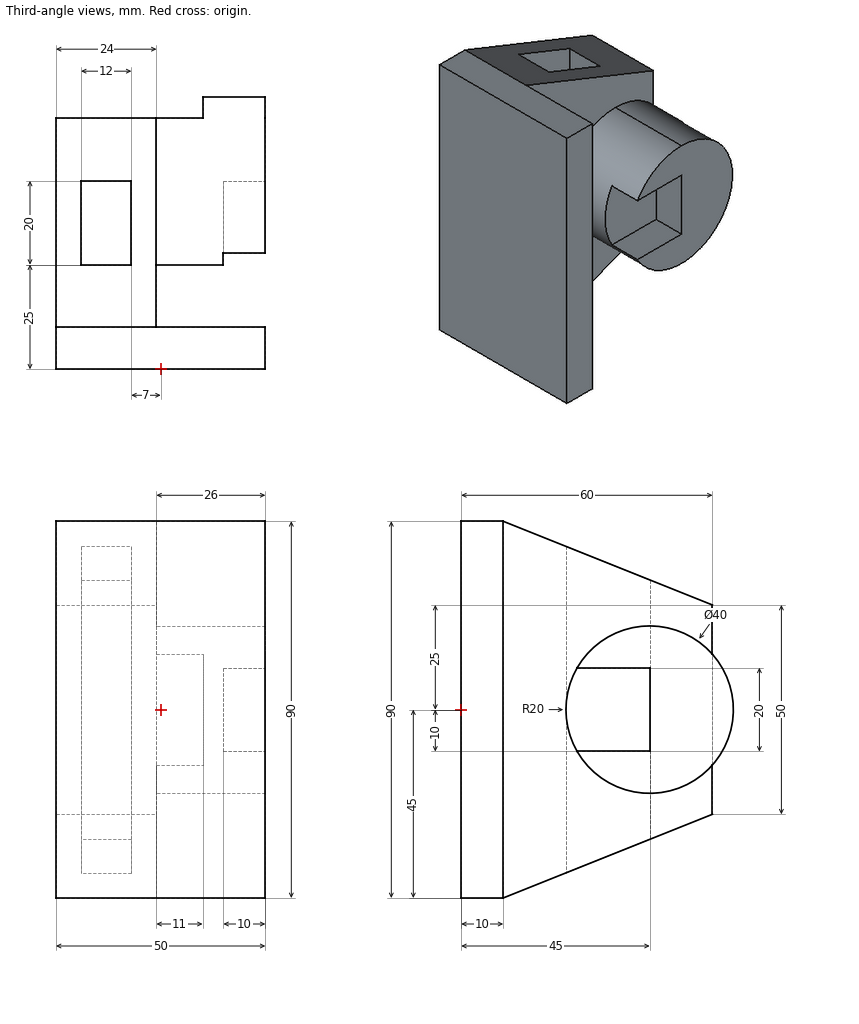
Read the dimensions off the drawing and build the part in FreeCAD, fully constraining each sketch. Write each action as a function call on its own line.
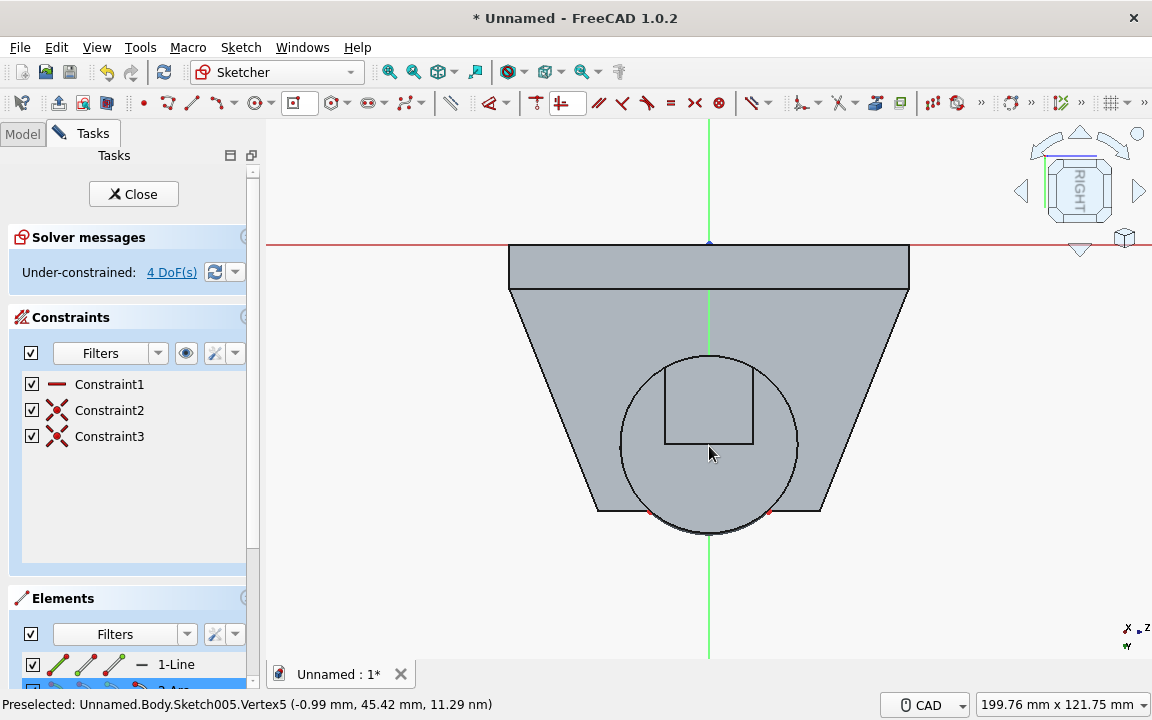
click(709, 596)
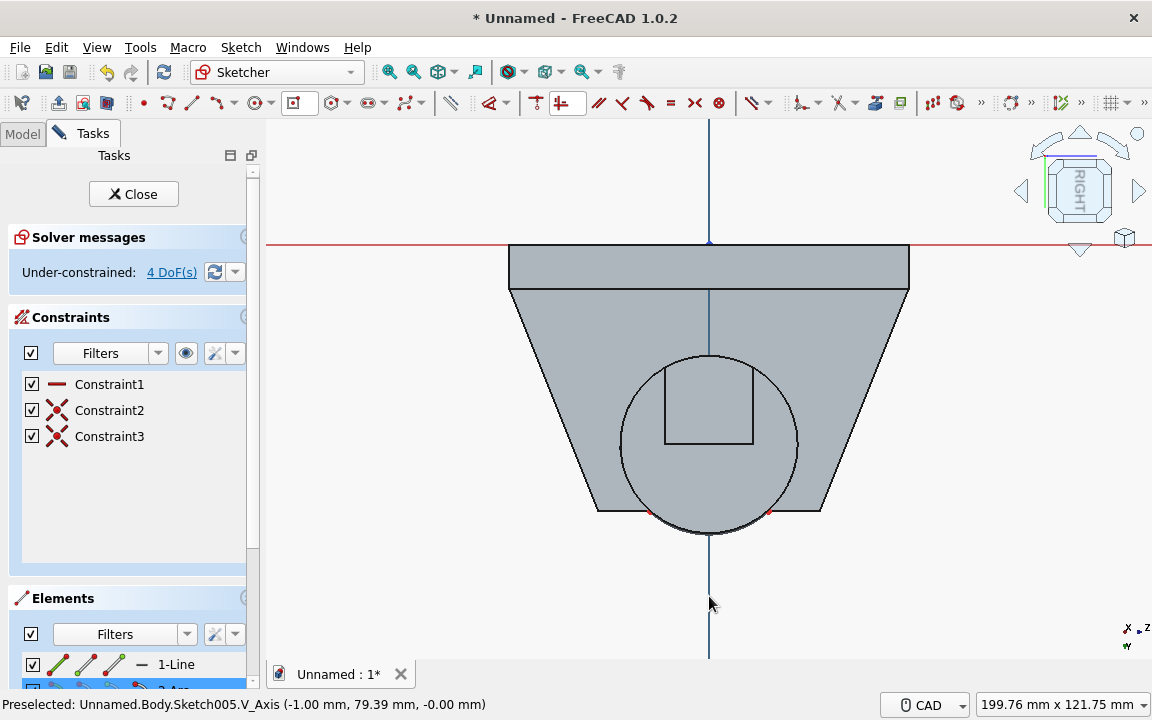
click(536, 104)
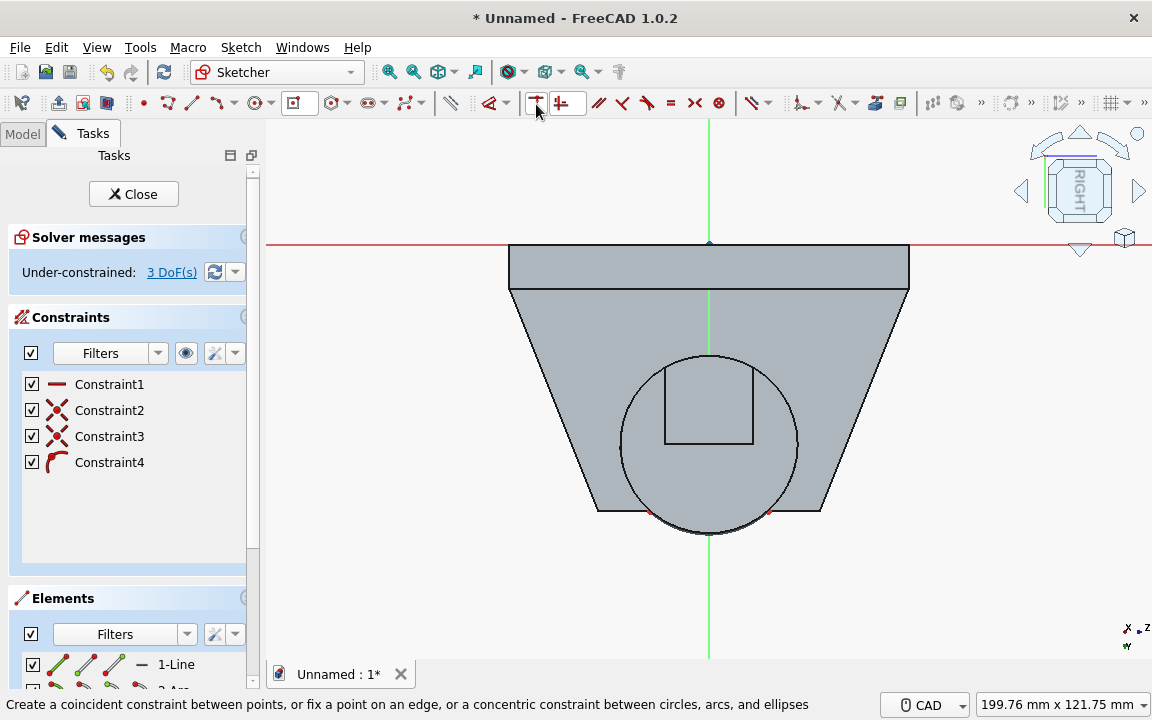
click(490, 104)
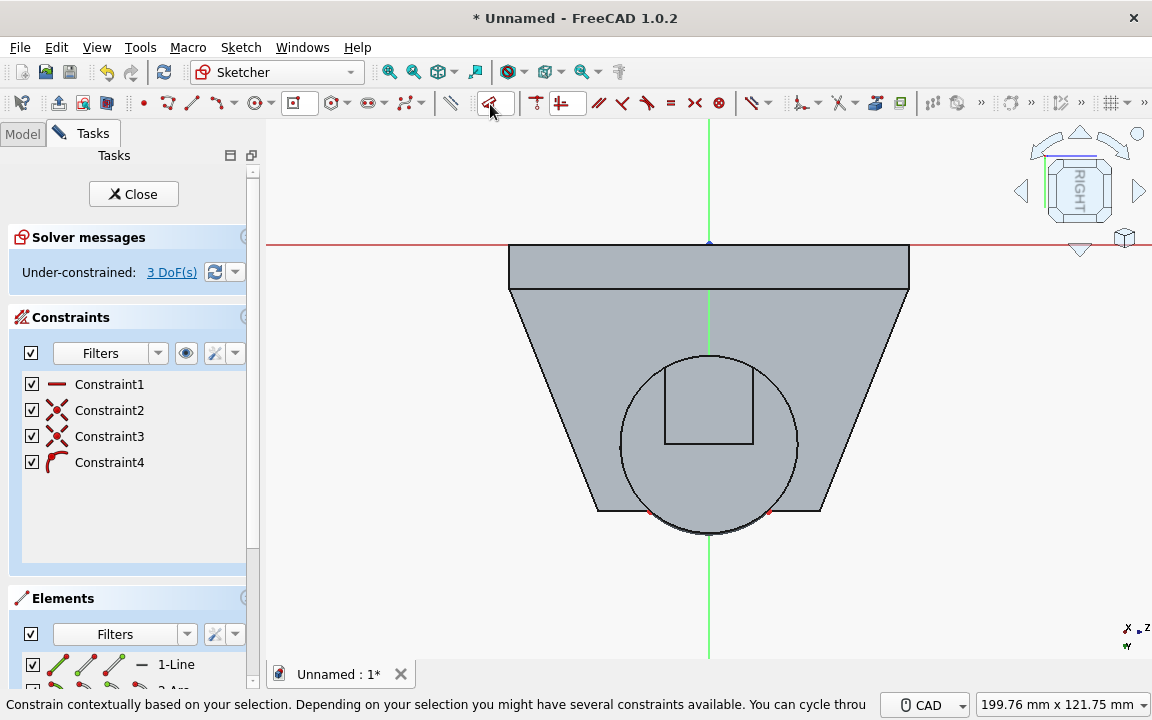
click(684, 531)
click(675, 562)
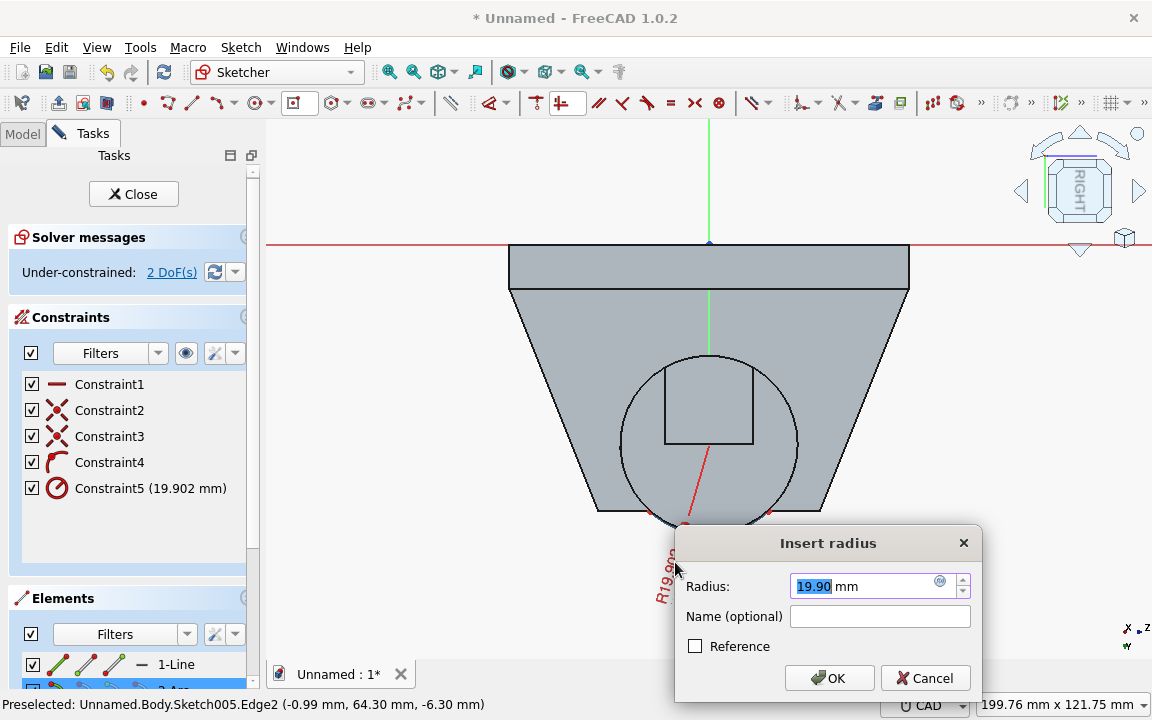
text(20)
key(Return)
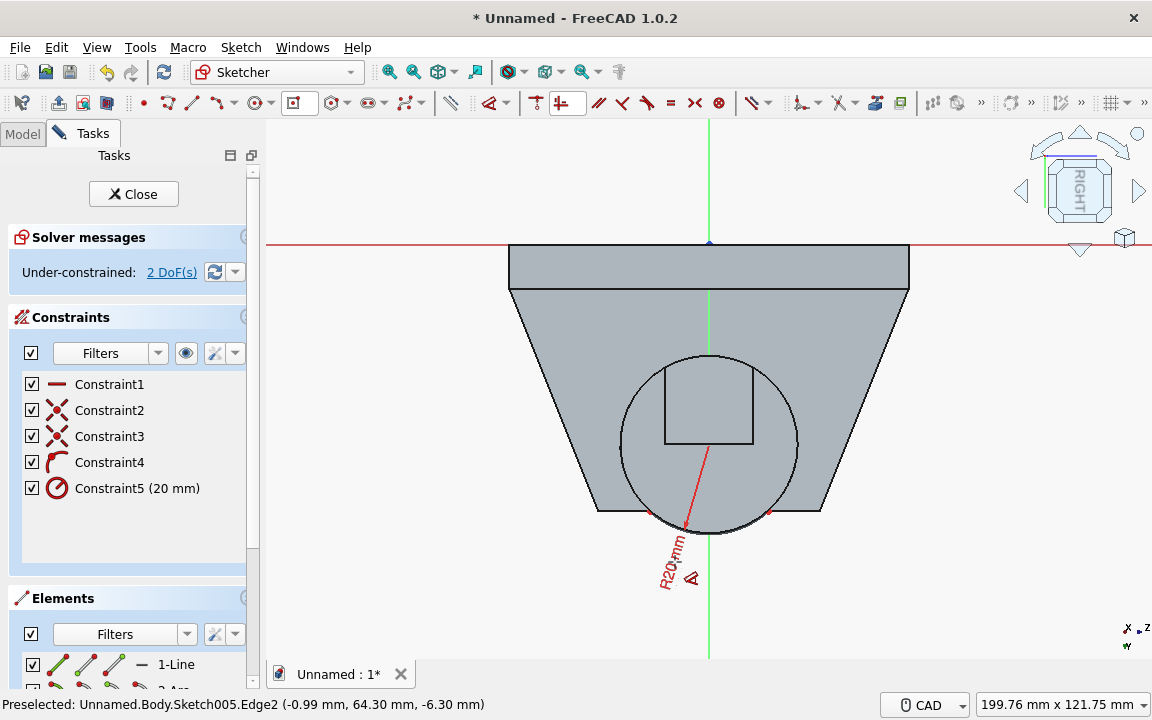
click(650, 512)
click(616, 378)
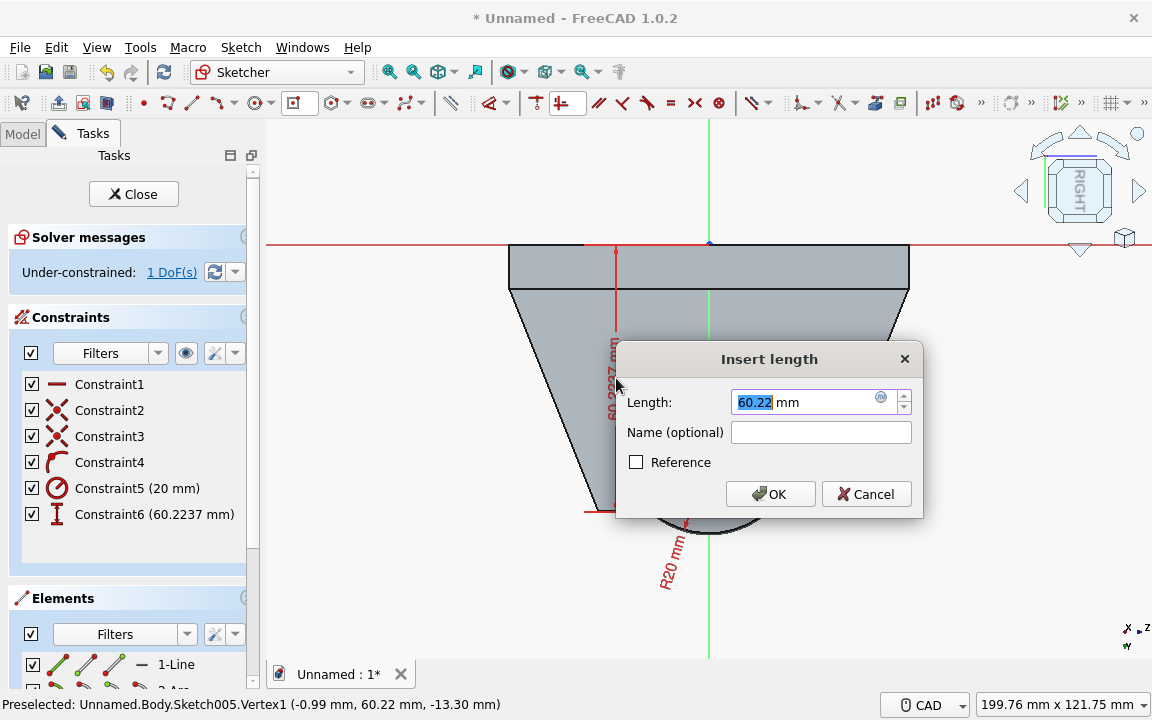
text(60)
key(Return)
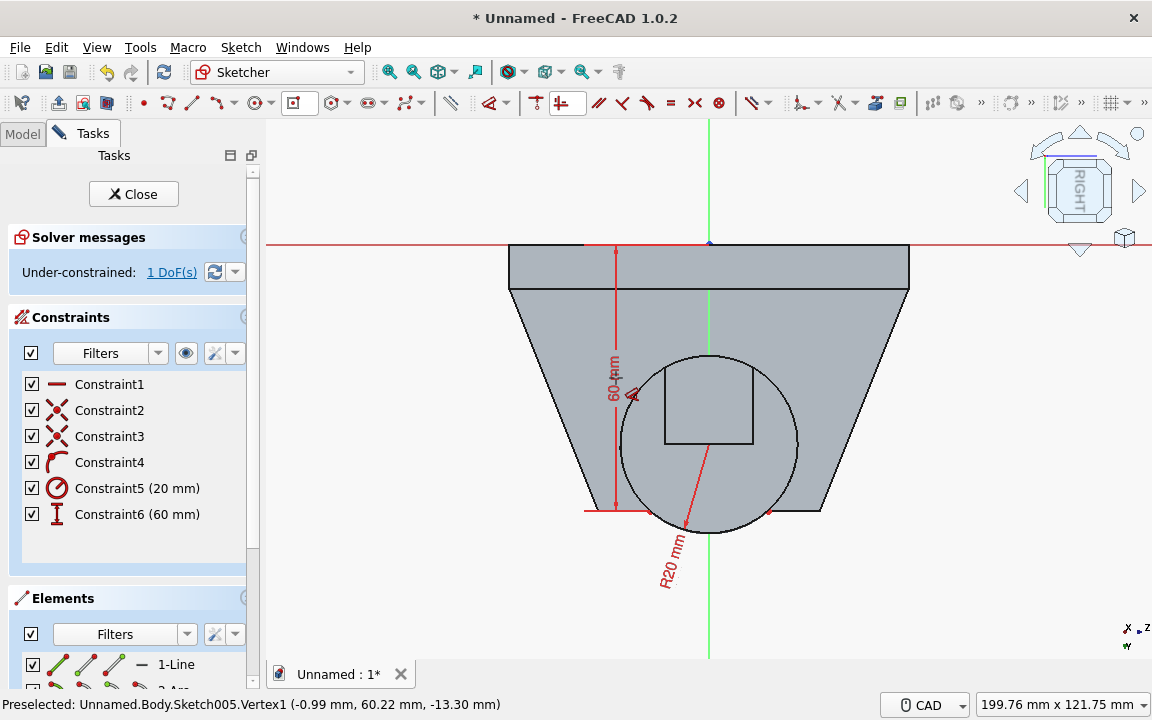
click(709, 445)
click(743, 345)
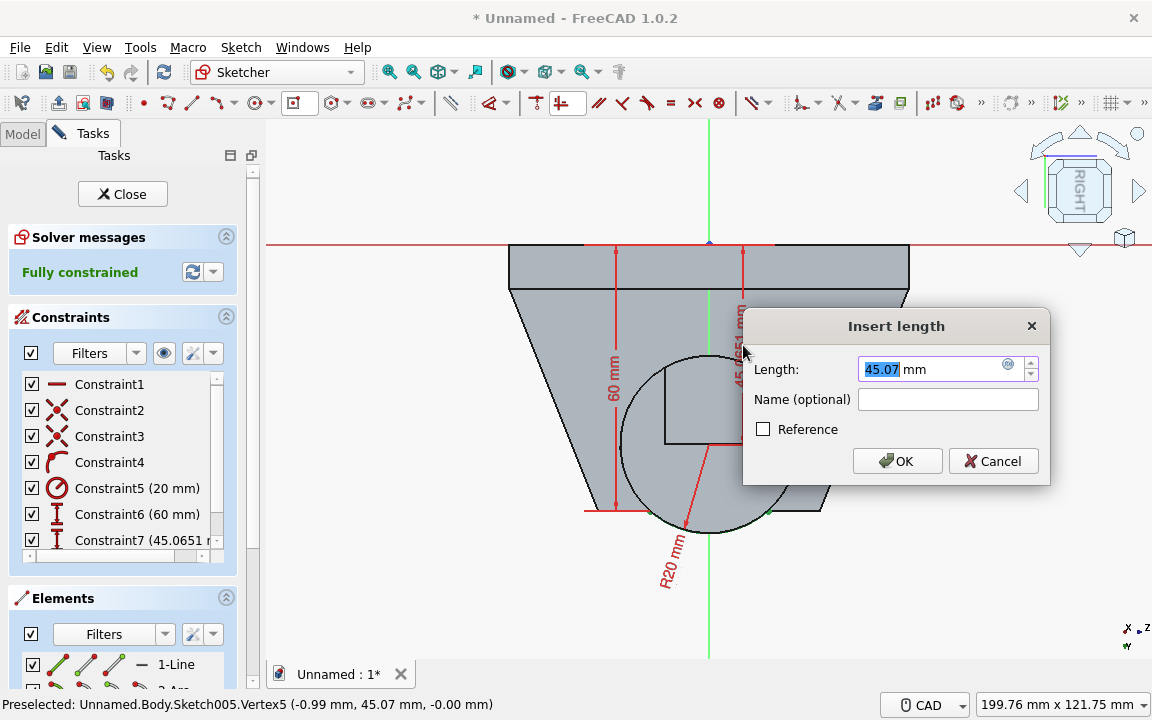
text(45)
key(Return)
key(Escape)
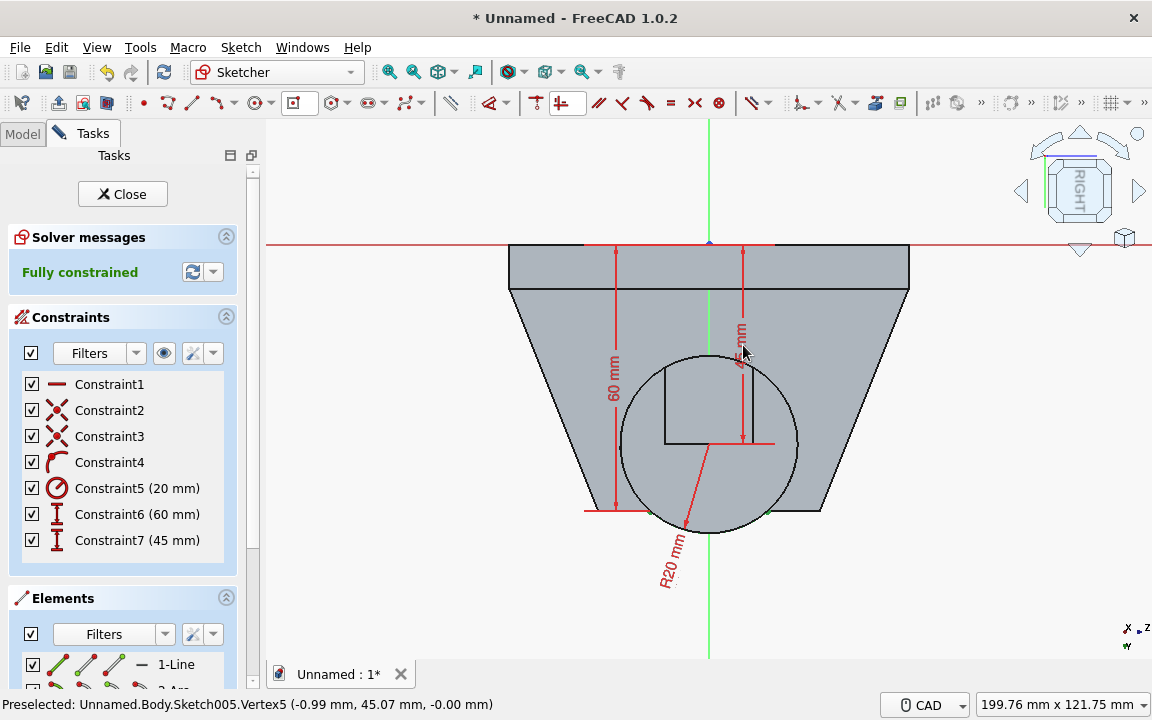
click(123, 194)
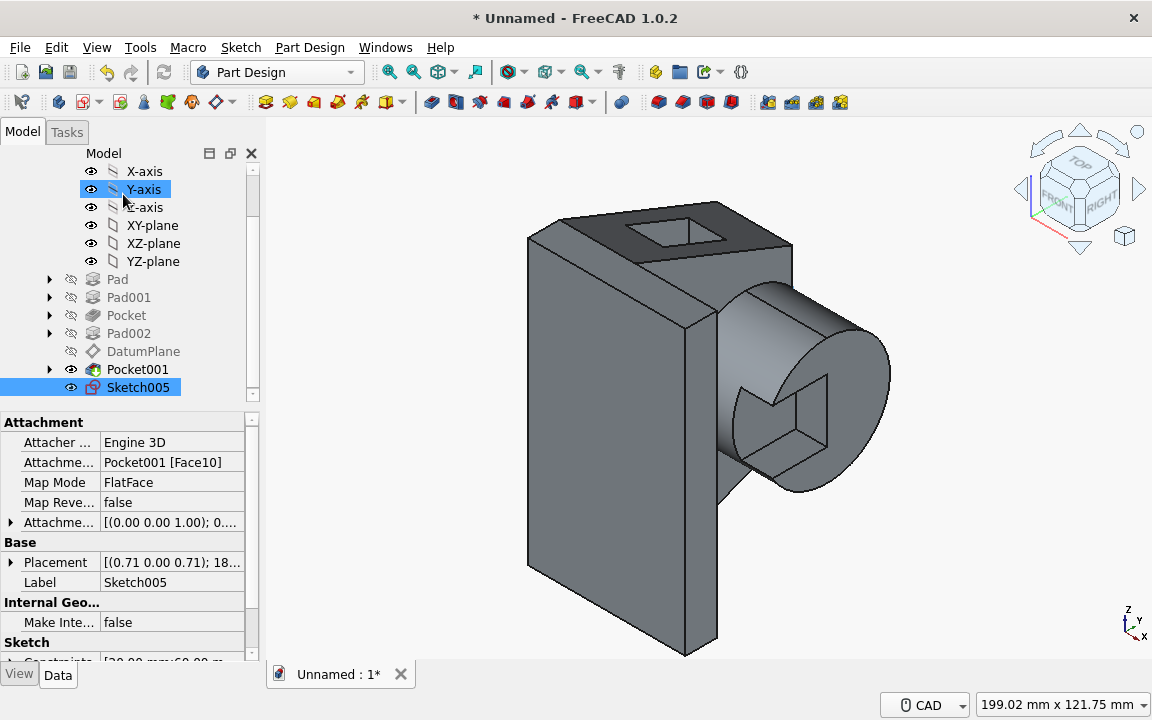
click(432, 102)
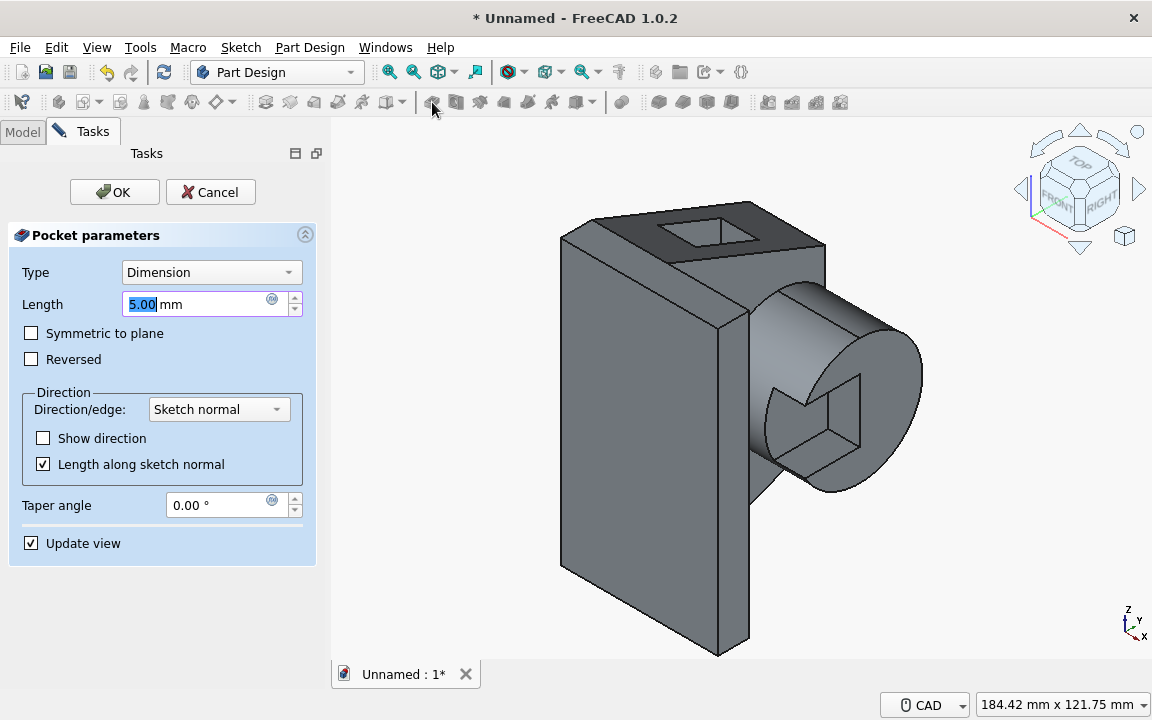
text(11)
key(Tab)